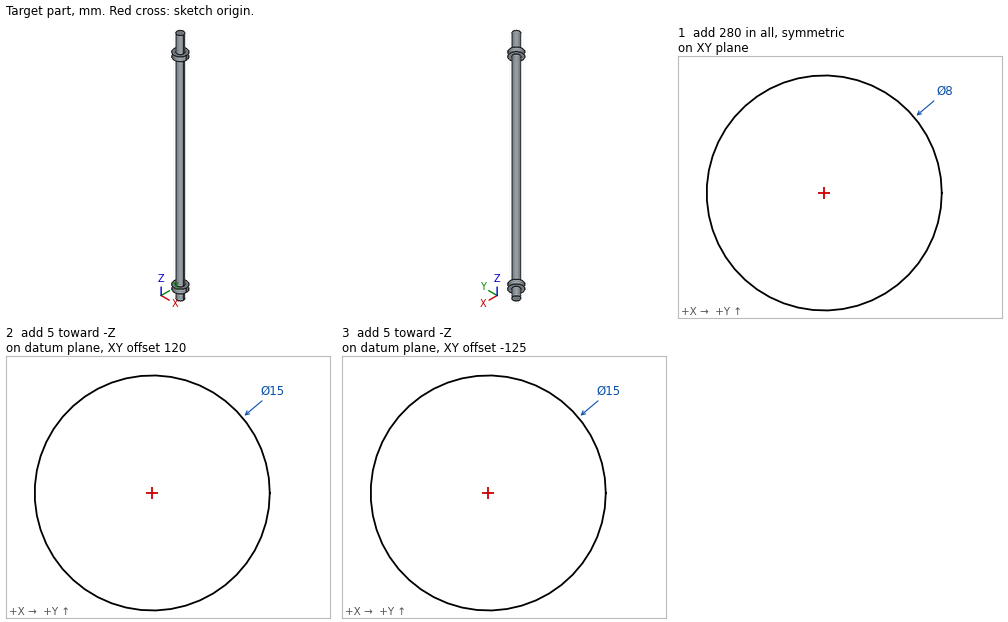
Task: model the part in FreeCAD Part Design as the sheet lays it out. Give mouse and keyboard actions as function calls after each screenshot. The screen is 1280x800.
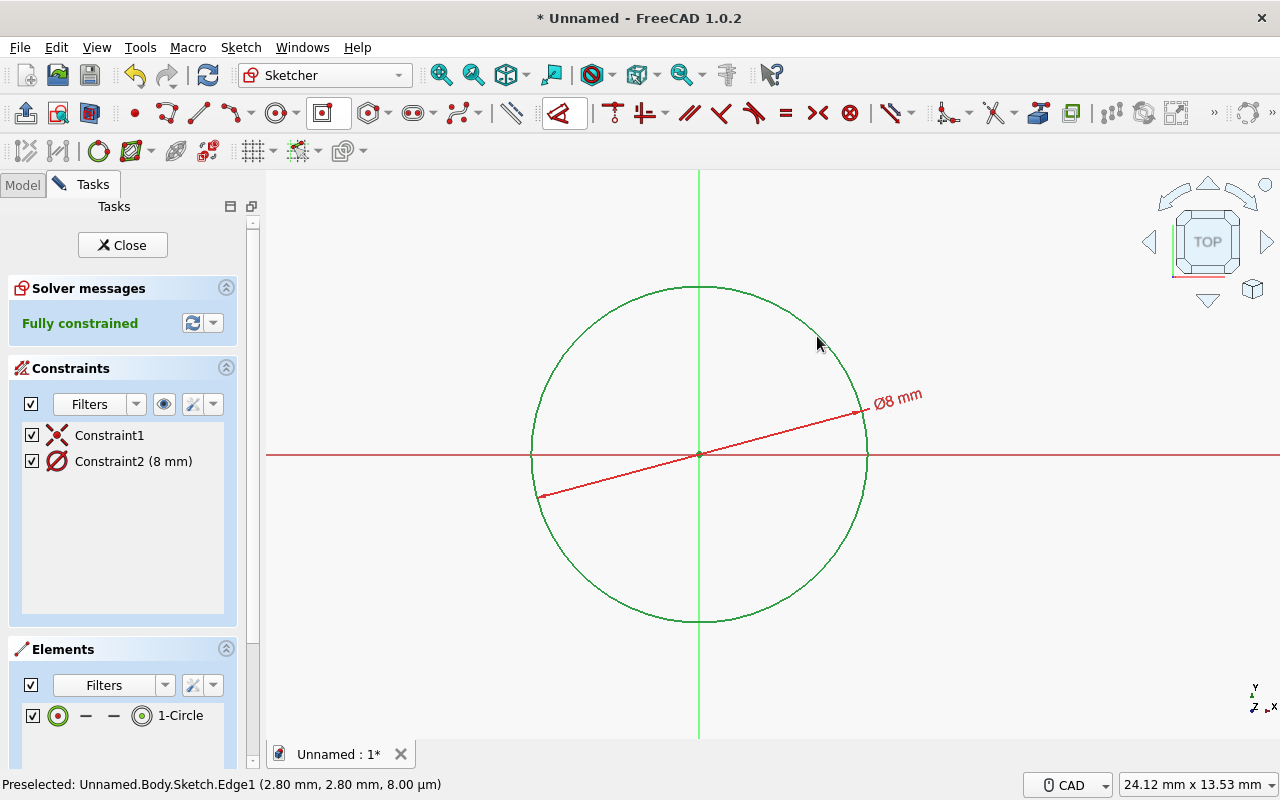
click(123, 245)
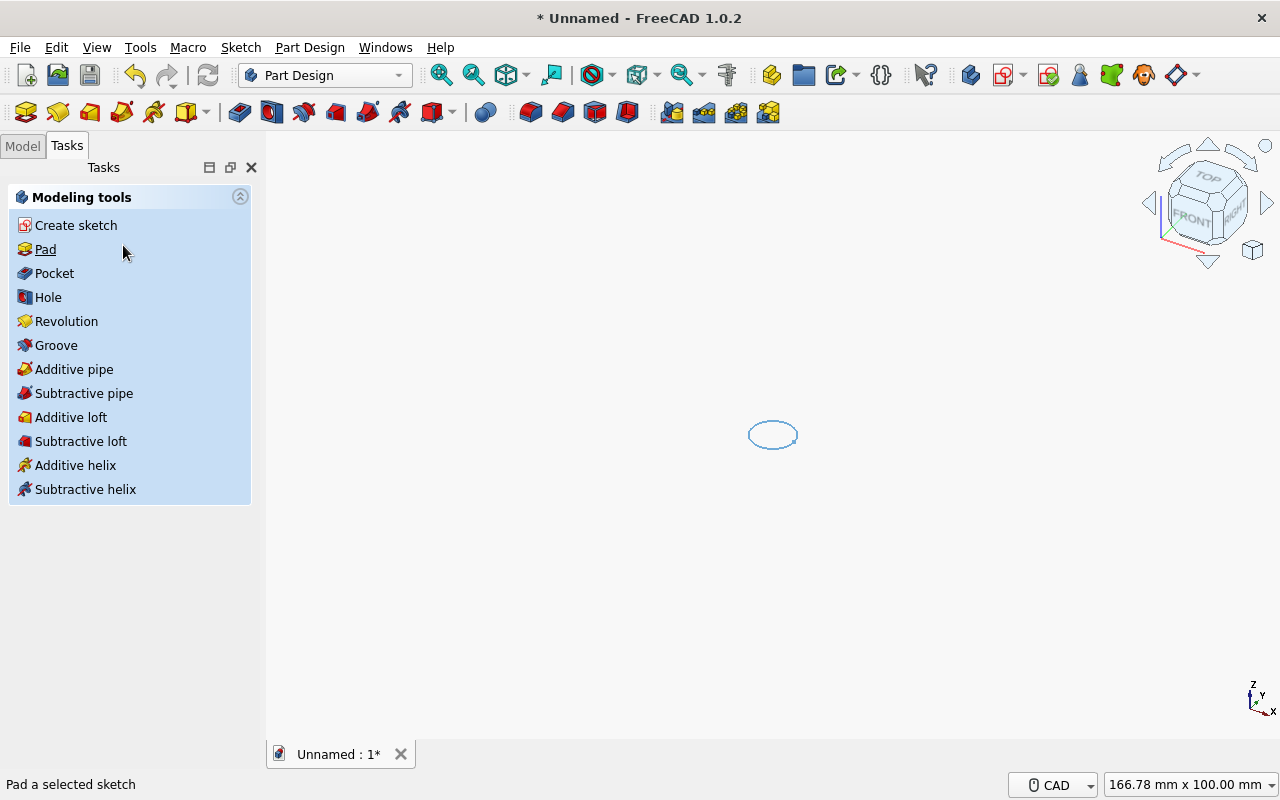
click(26, 112)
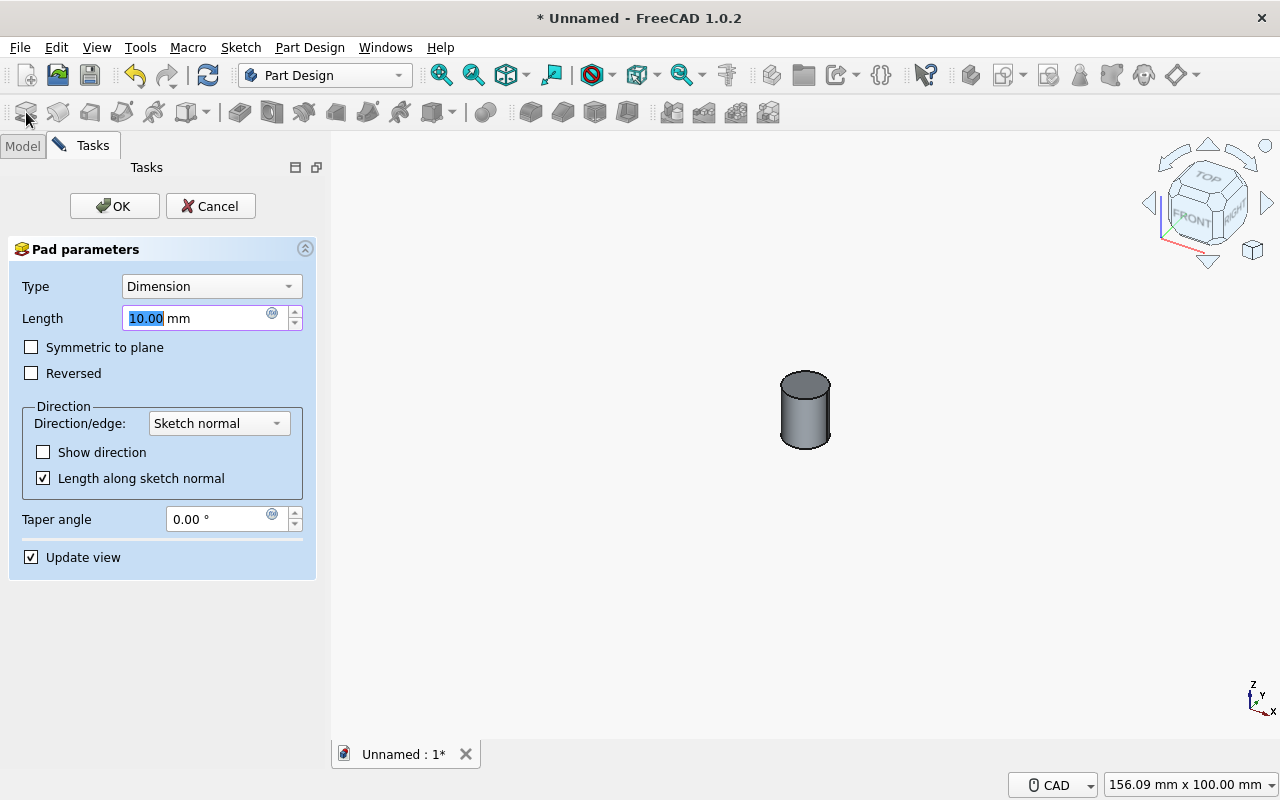
text(280)
key(Tab)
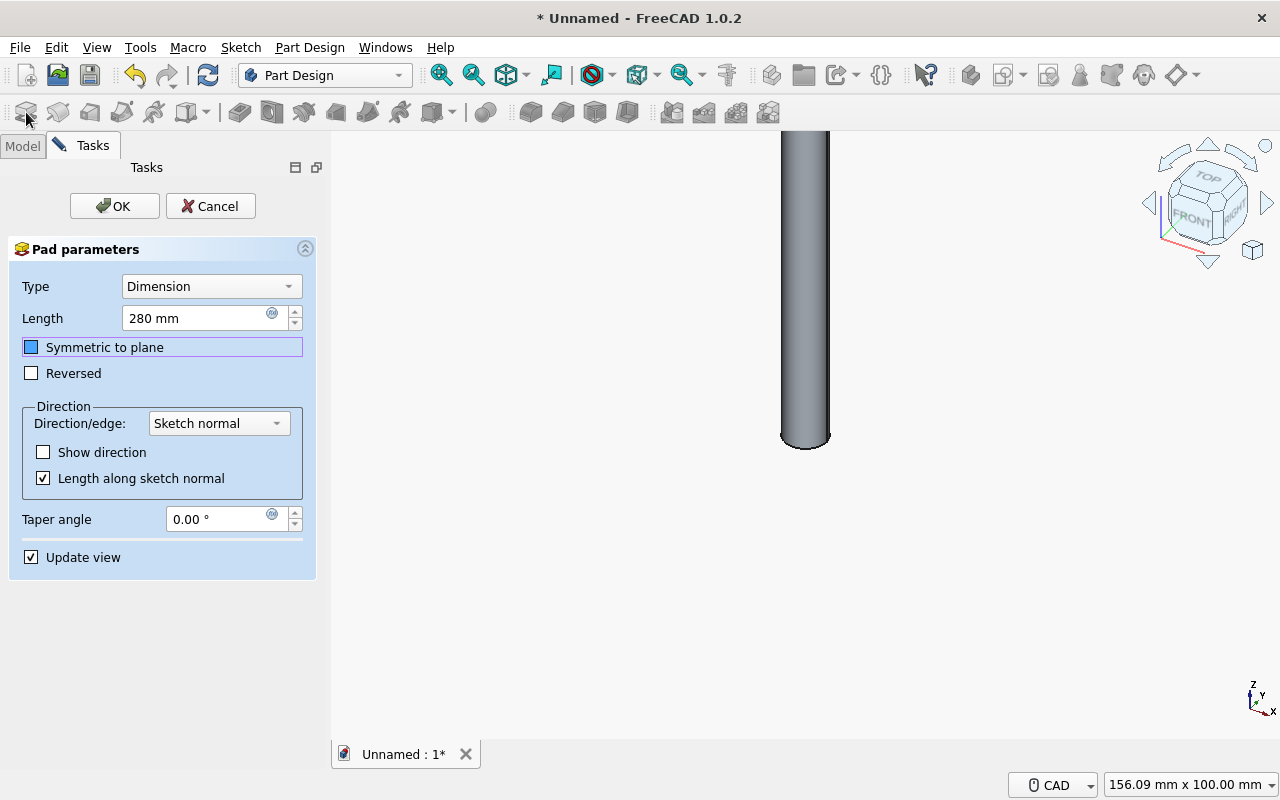
click(30, 347)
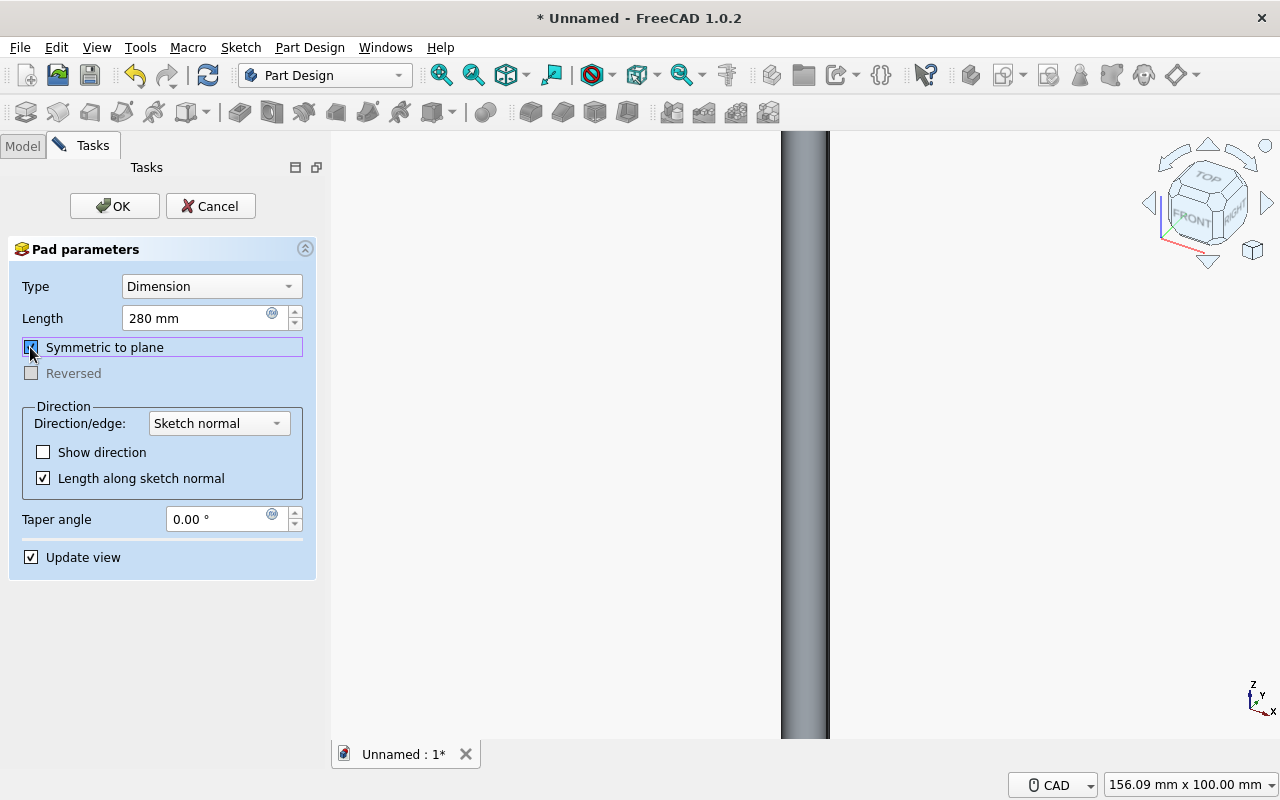
click(115, 206)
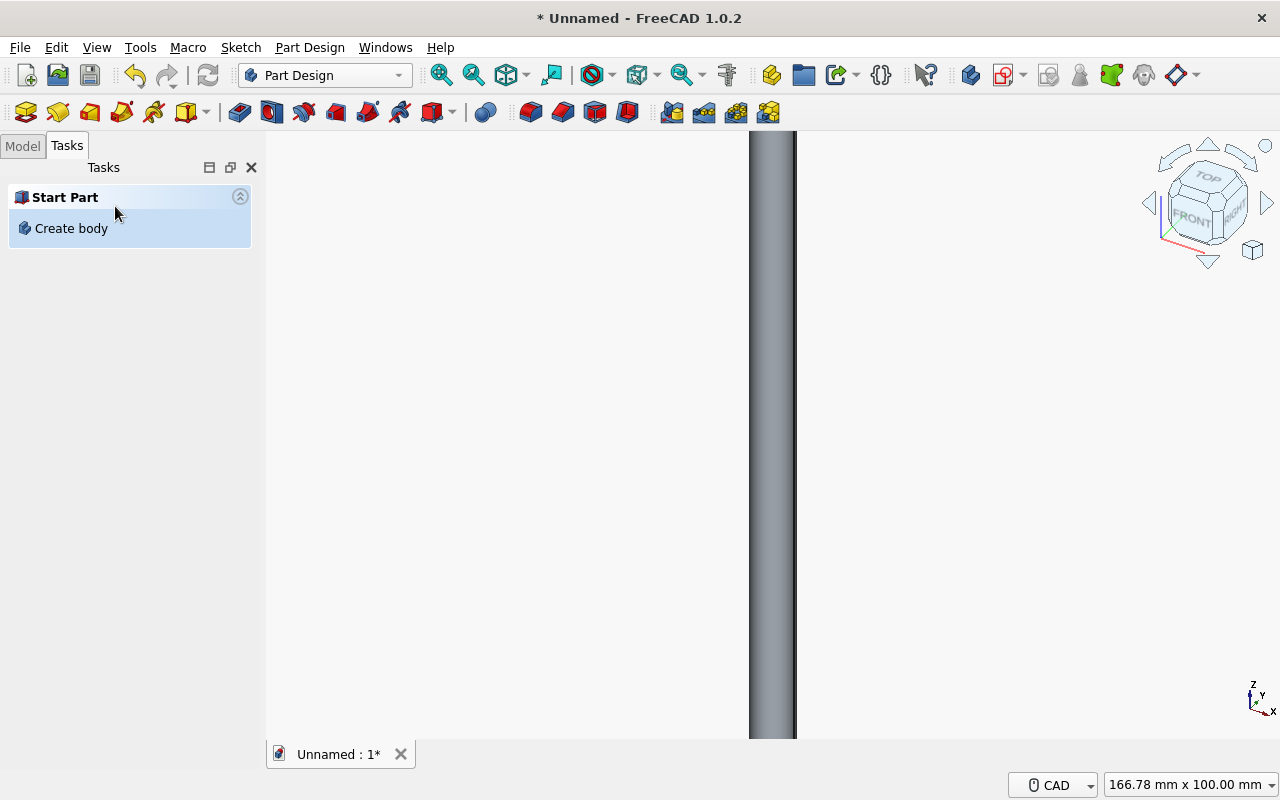
click(442, 76)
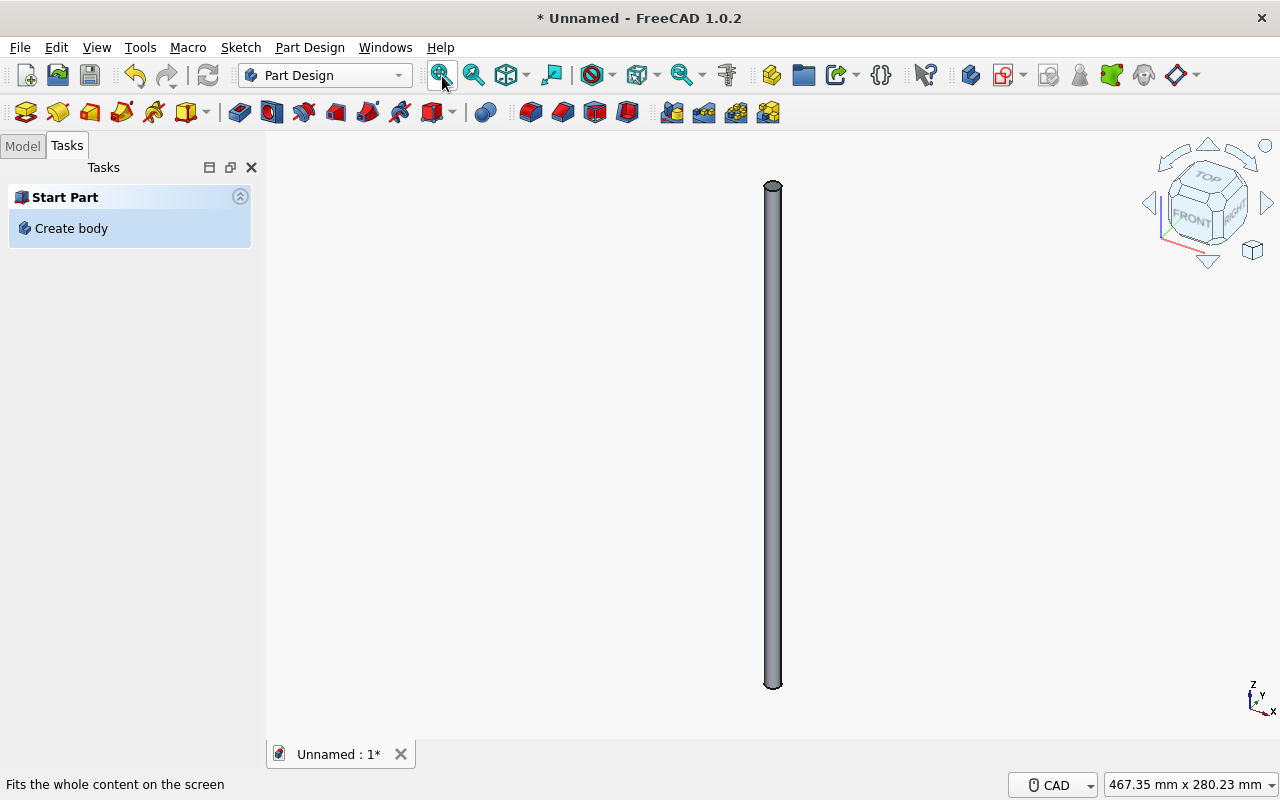
click(23, 145)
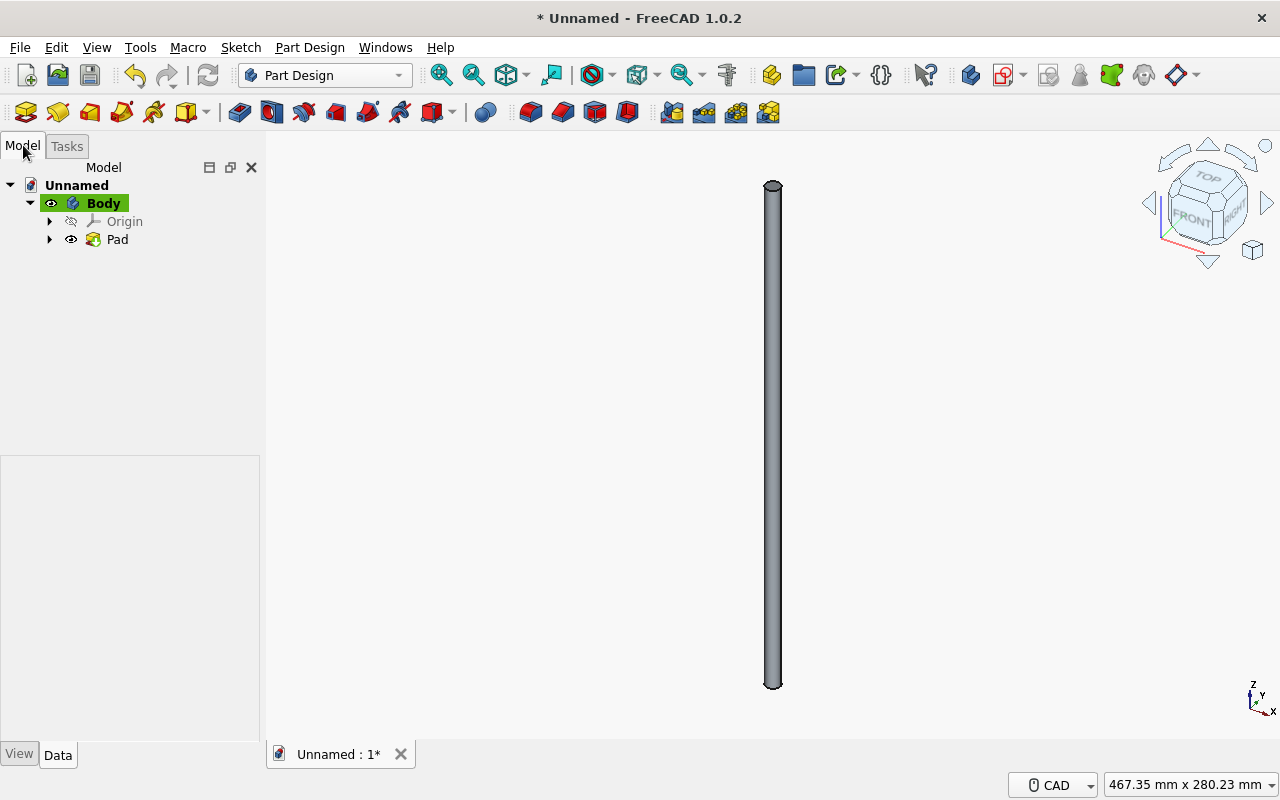
click(50, 221)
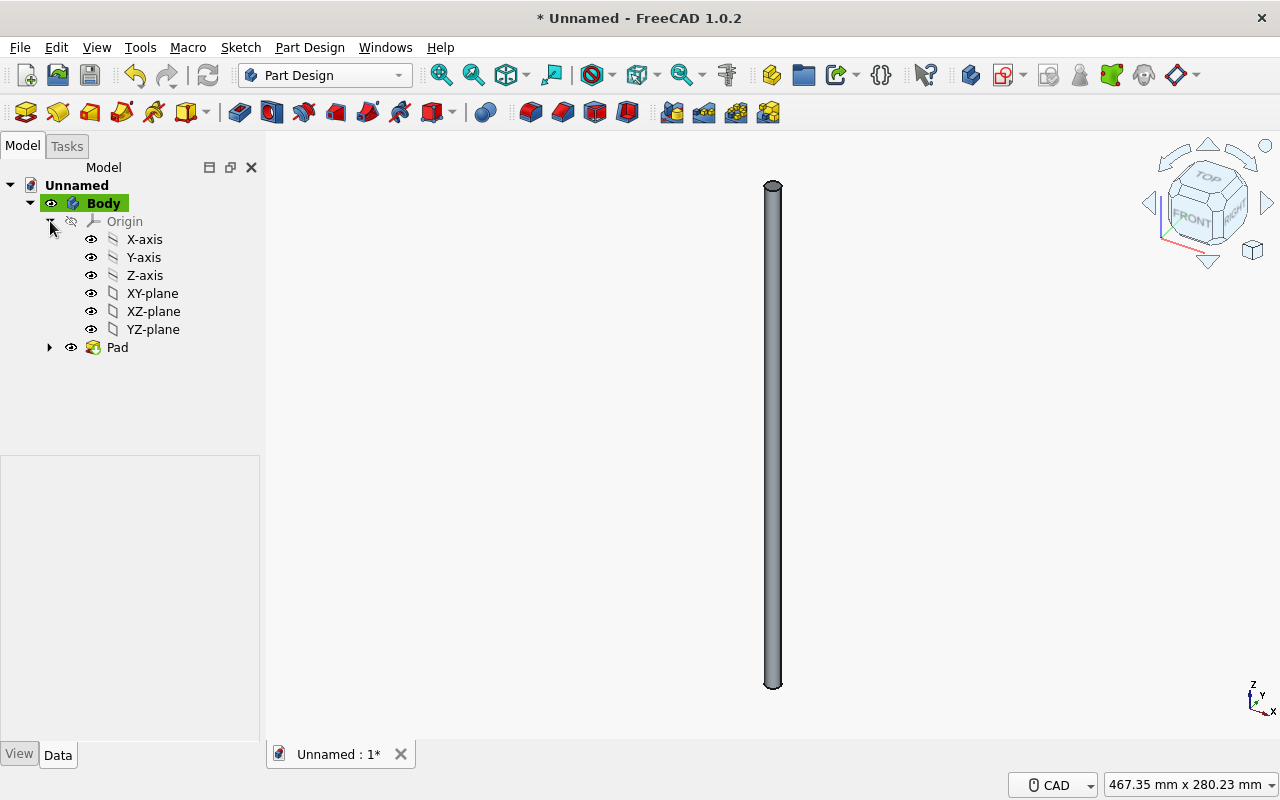
click(136, 293)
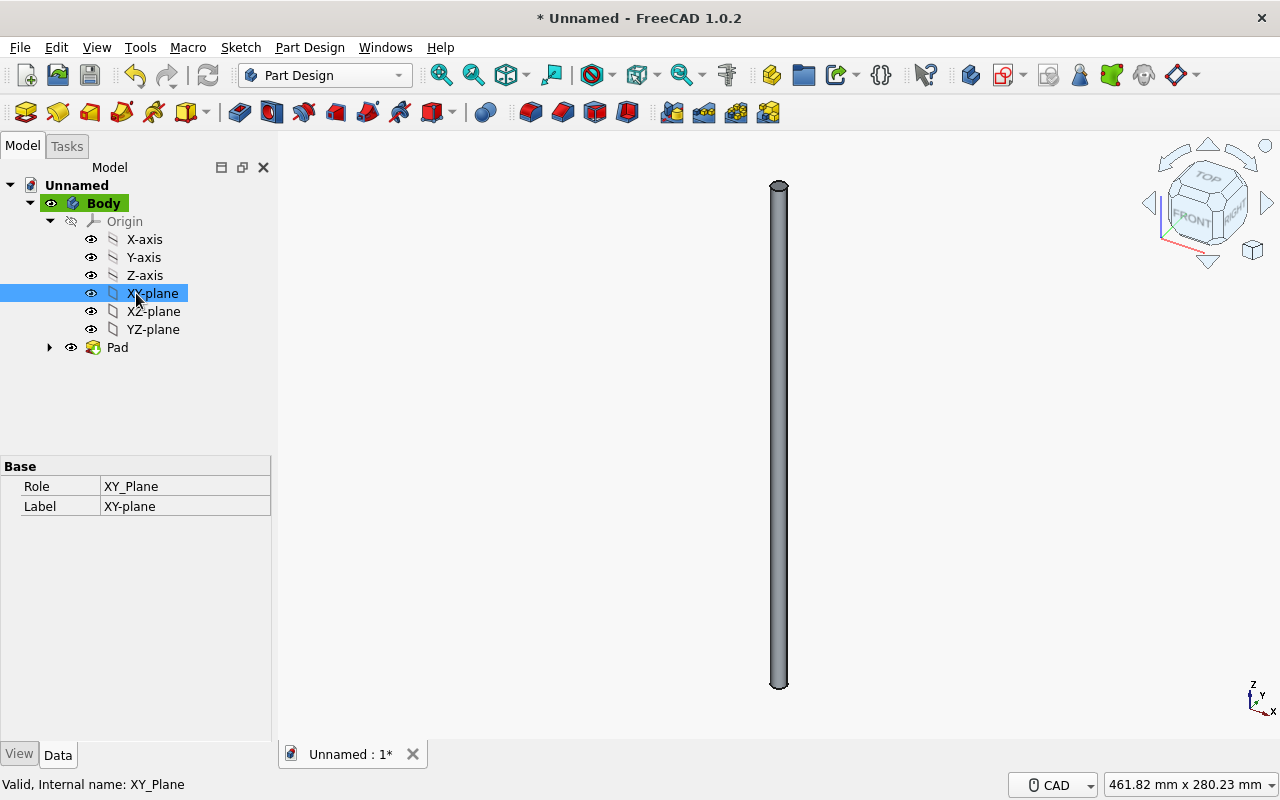
click(1176, 76)